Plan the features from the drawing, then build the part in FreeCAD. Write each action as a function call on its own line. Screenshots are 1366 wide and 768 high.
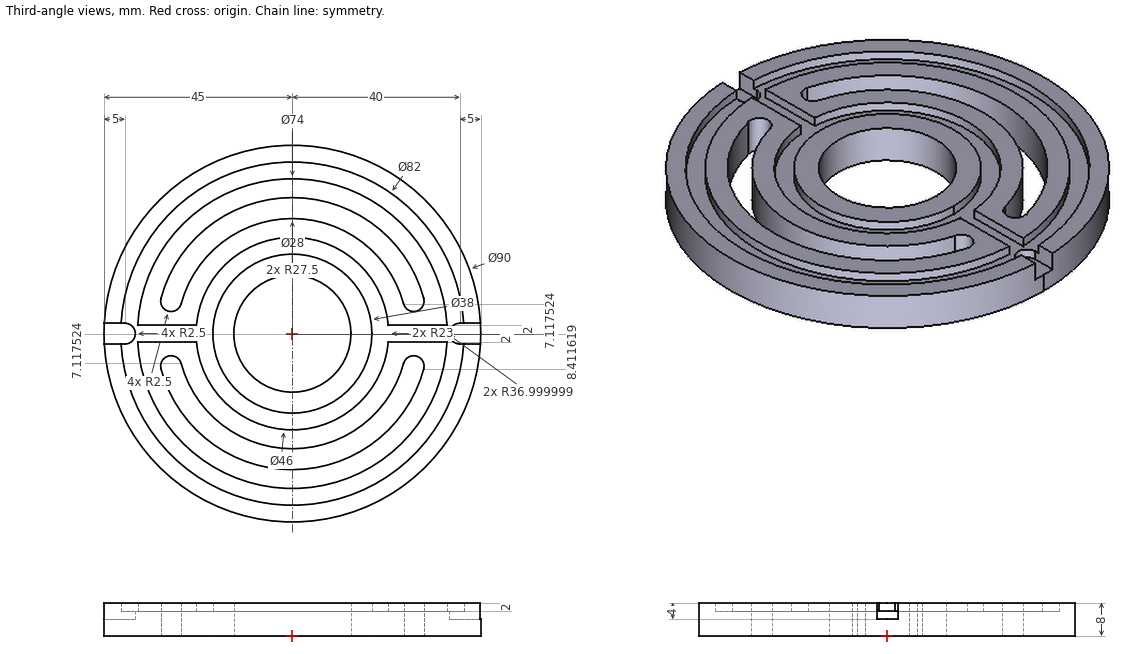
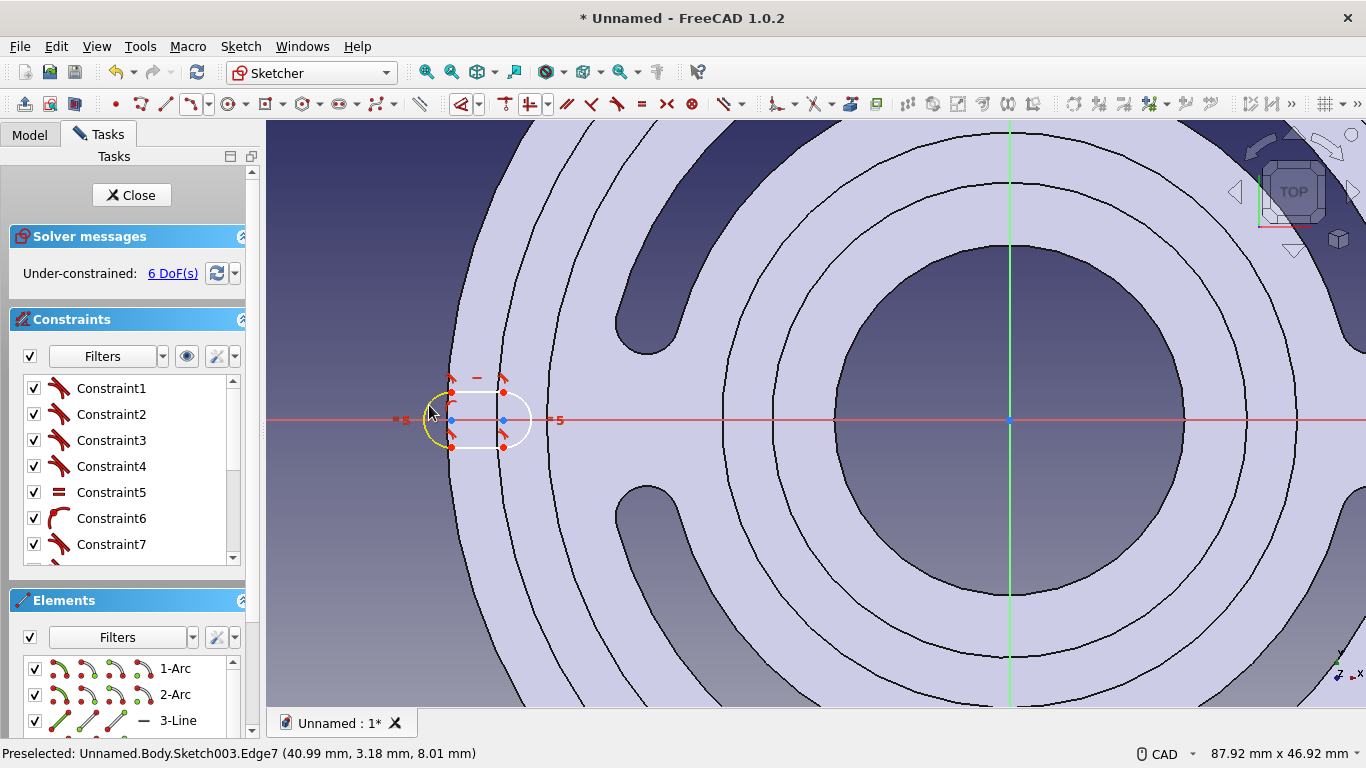
click(429, 404)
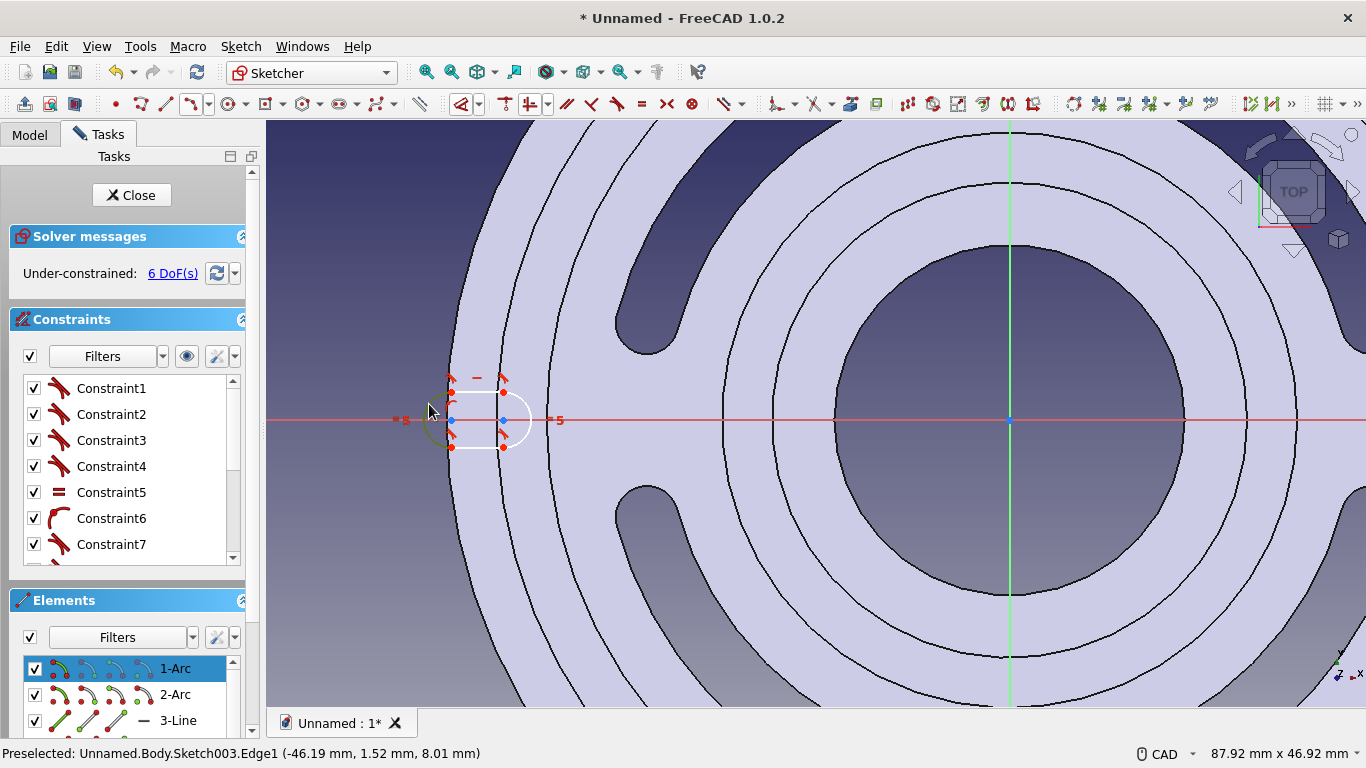
scroll(429, 405, down, 3)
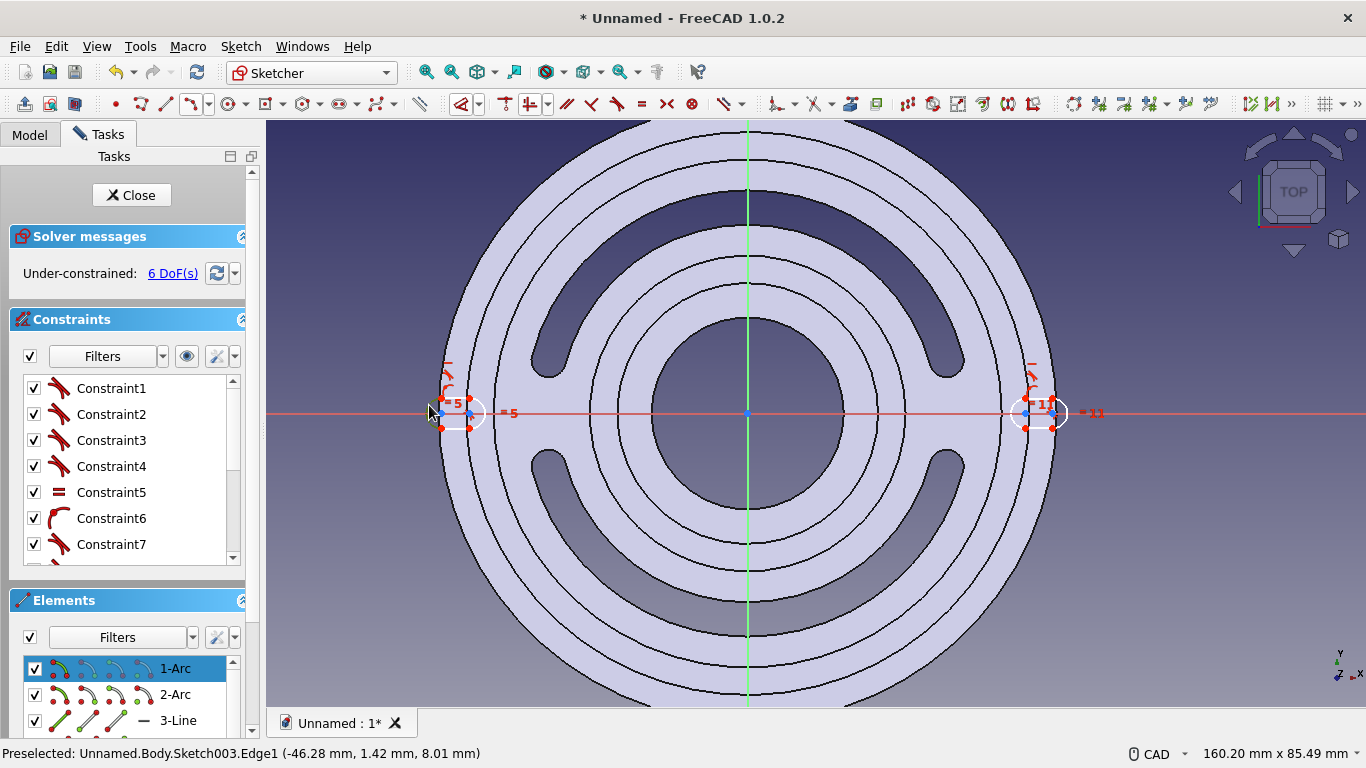
scroll(1014, 405, up, 3)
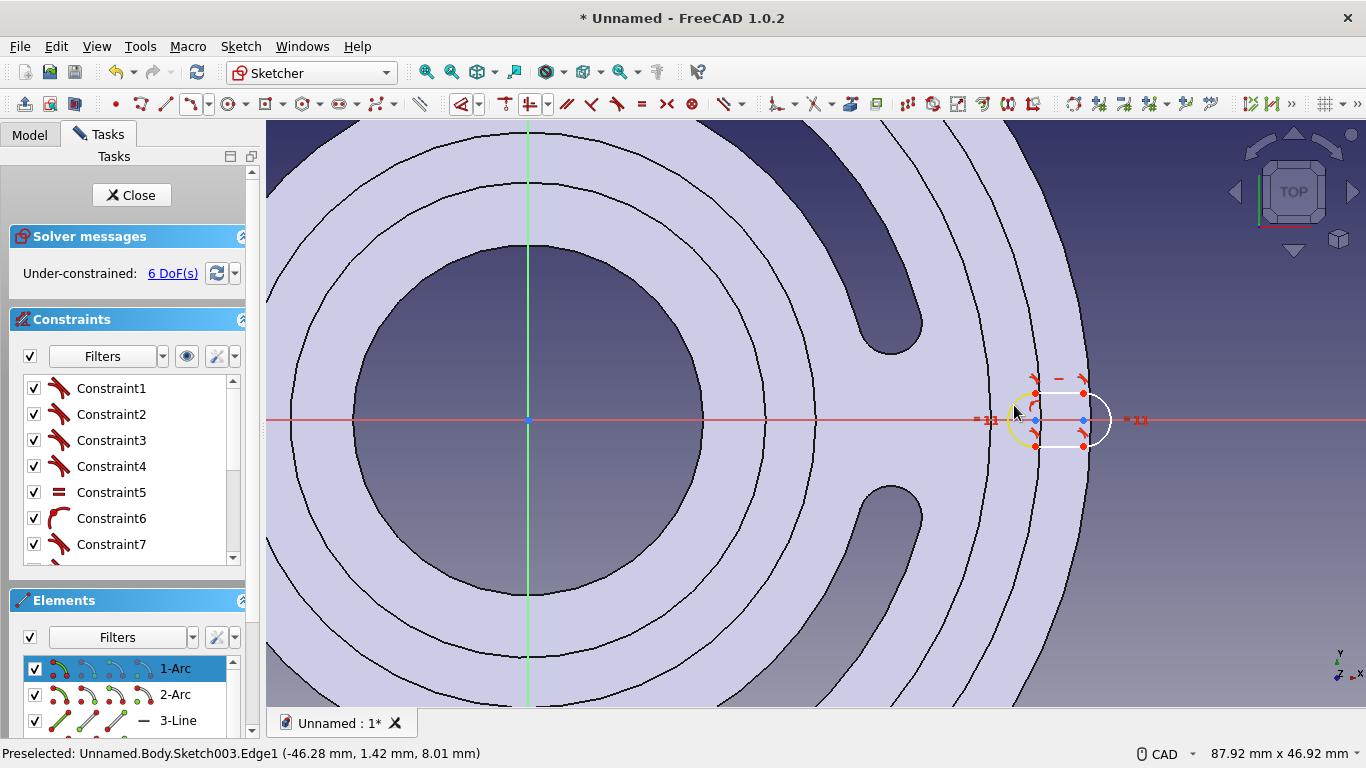
click(1013, 404)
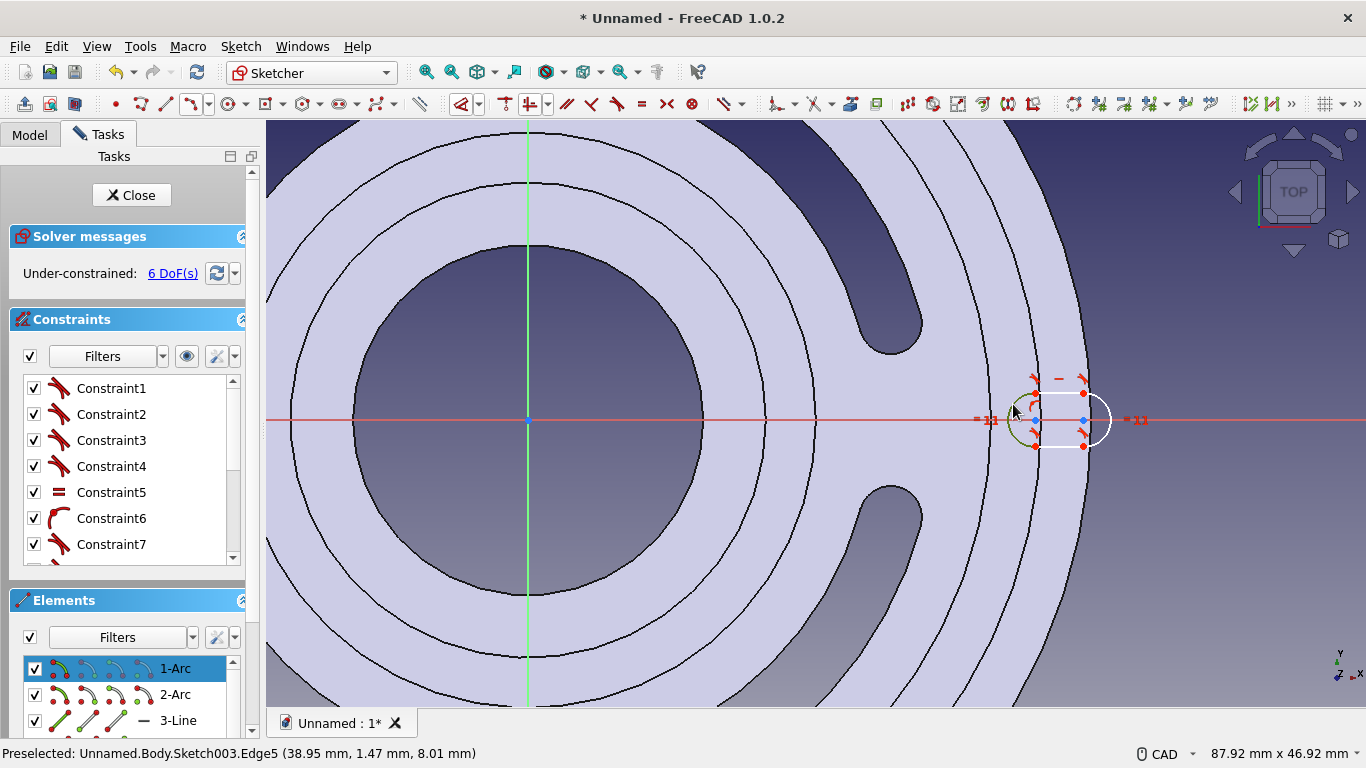
key(e)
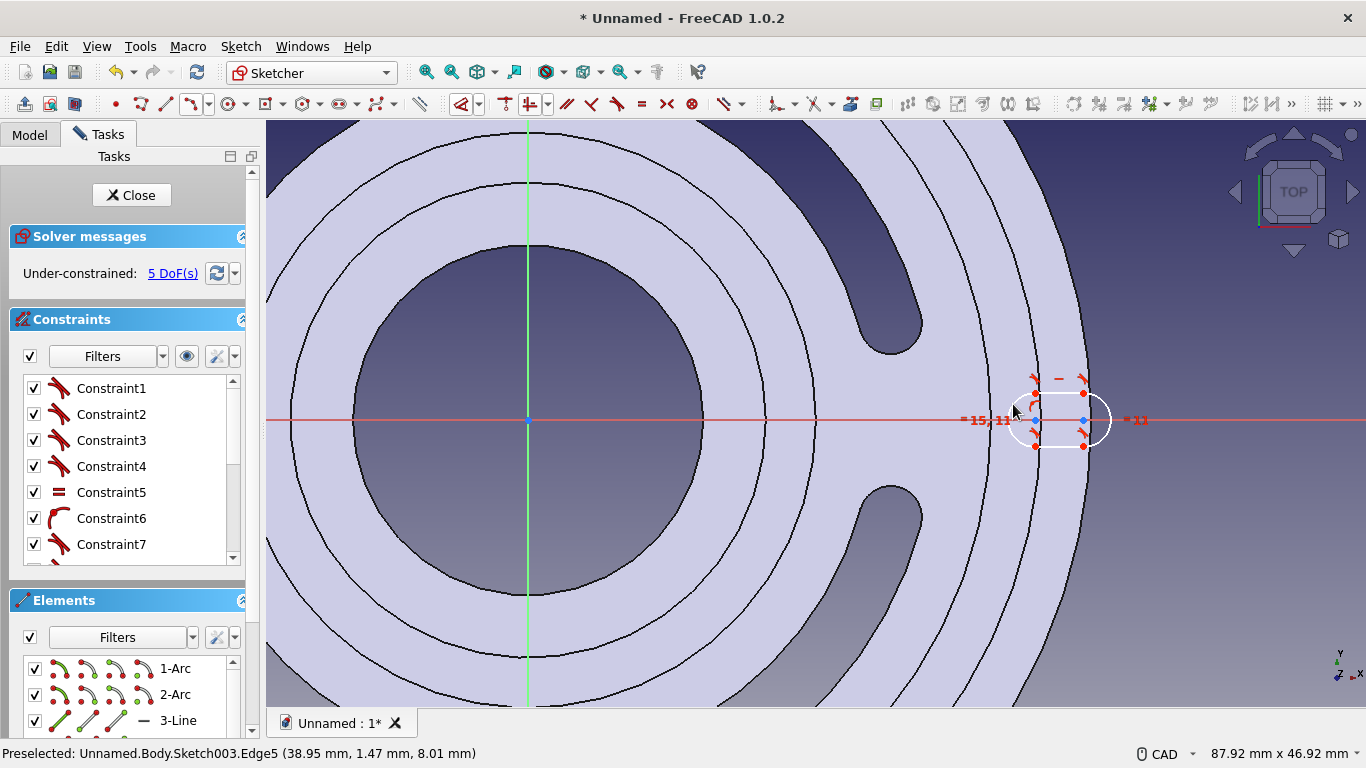
key(d)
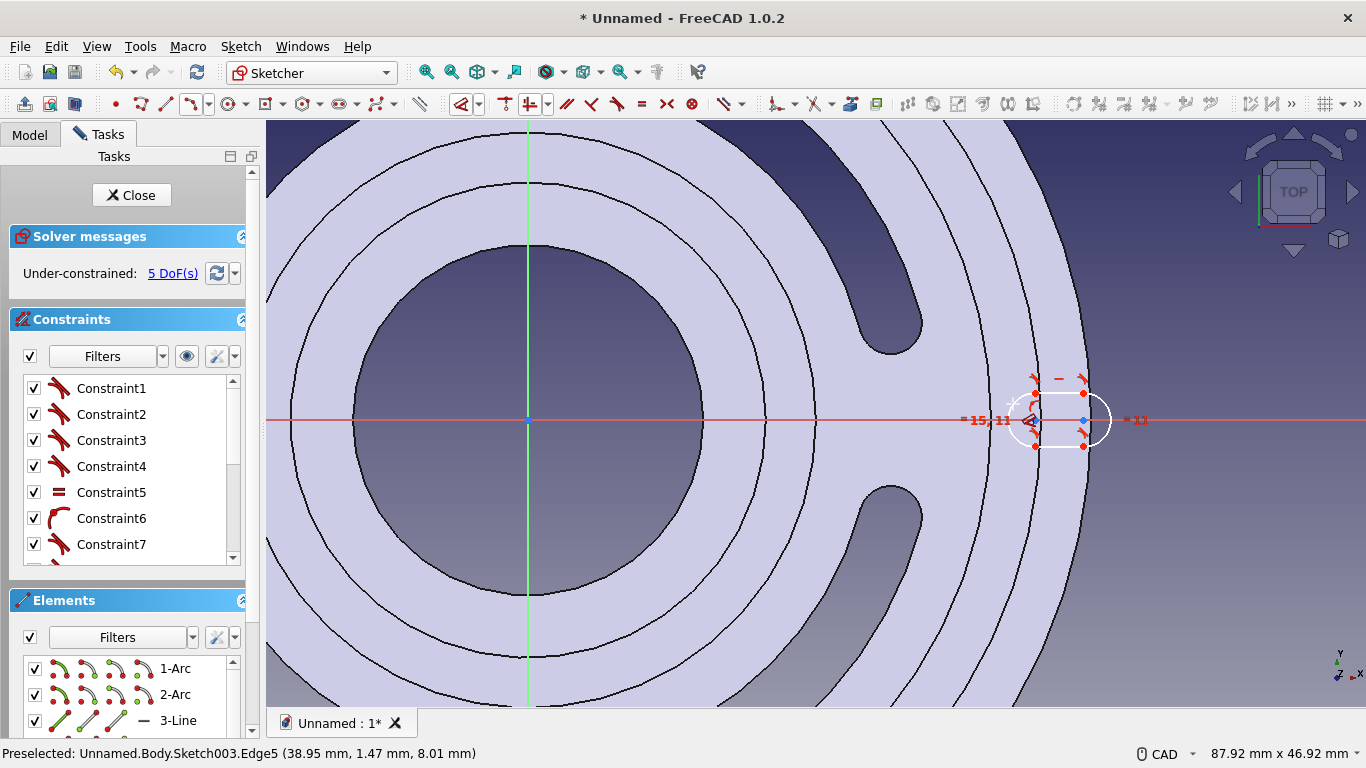
scroll(1014, 405, down, 3)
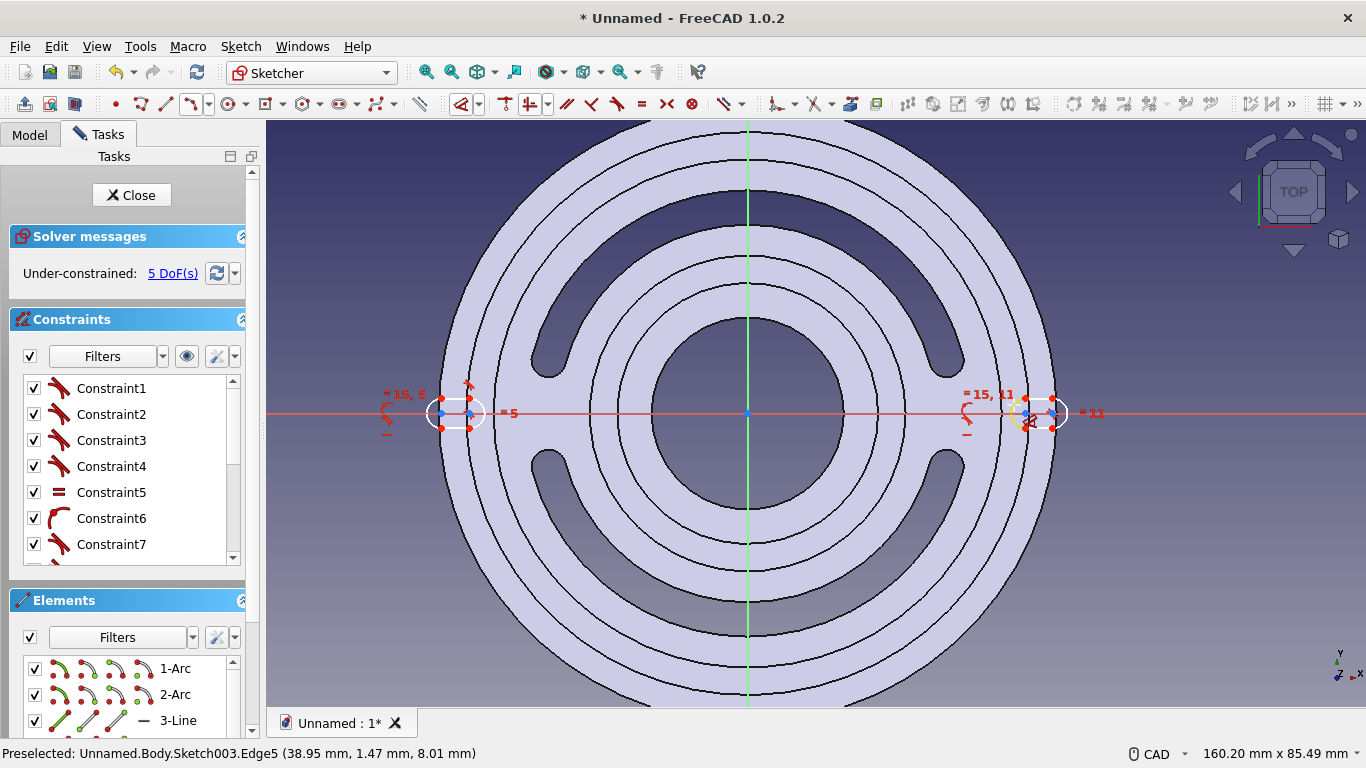
scroll(430, 405, up, 5)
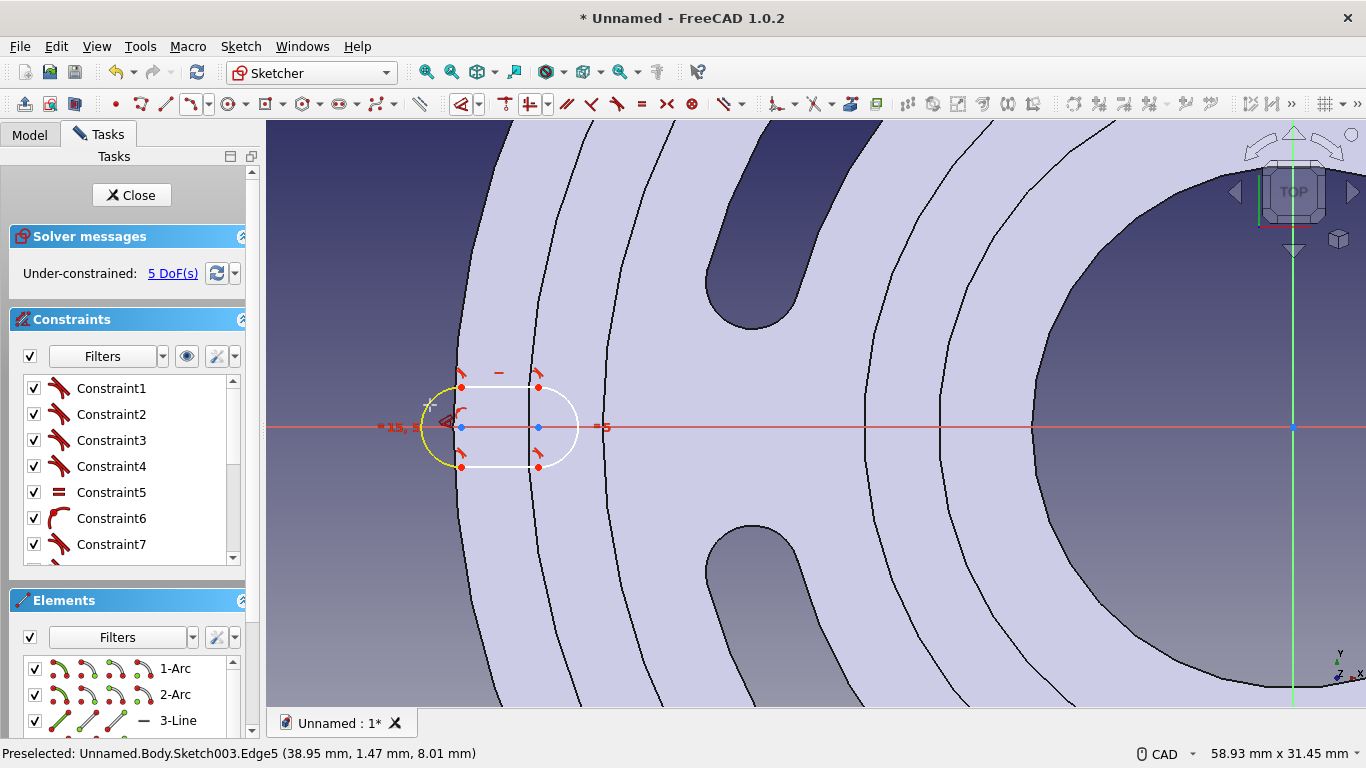
click(429, 404)
click(403, 385)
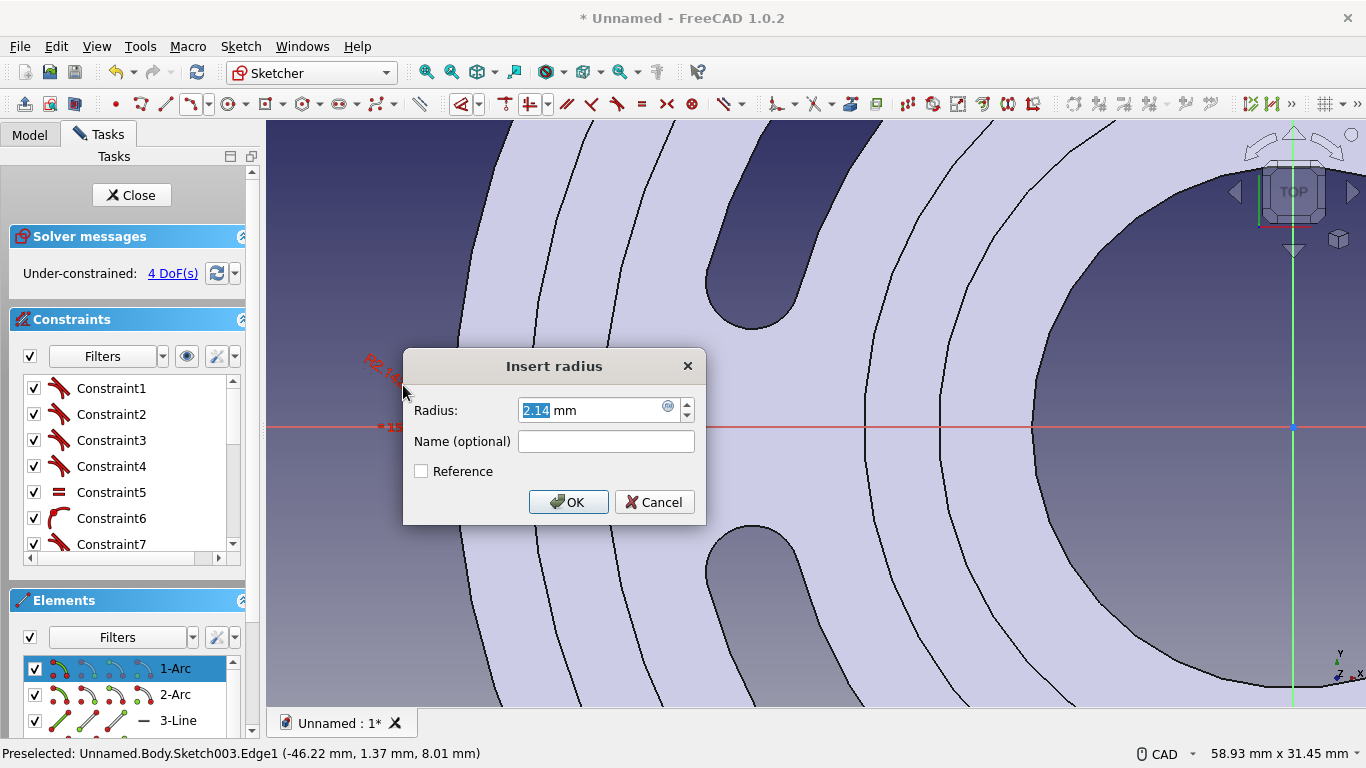
text(2.5)
key(Return)